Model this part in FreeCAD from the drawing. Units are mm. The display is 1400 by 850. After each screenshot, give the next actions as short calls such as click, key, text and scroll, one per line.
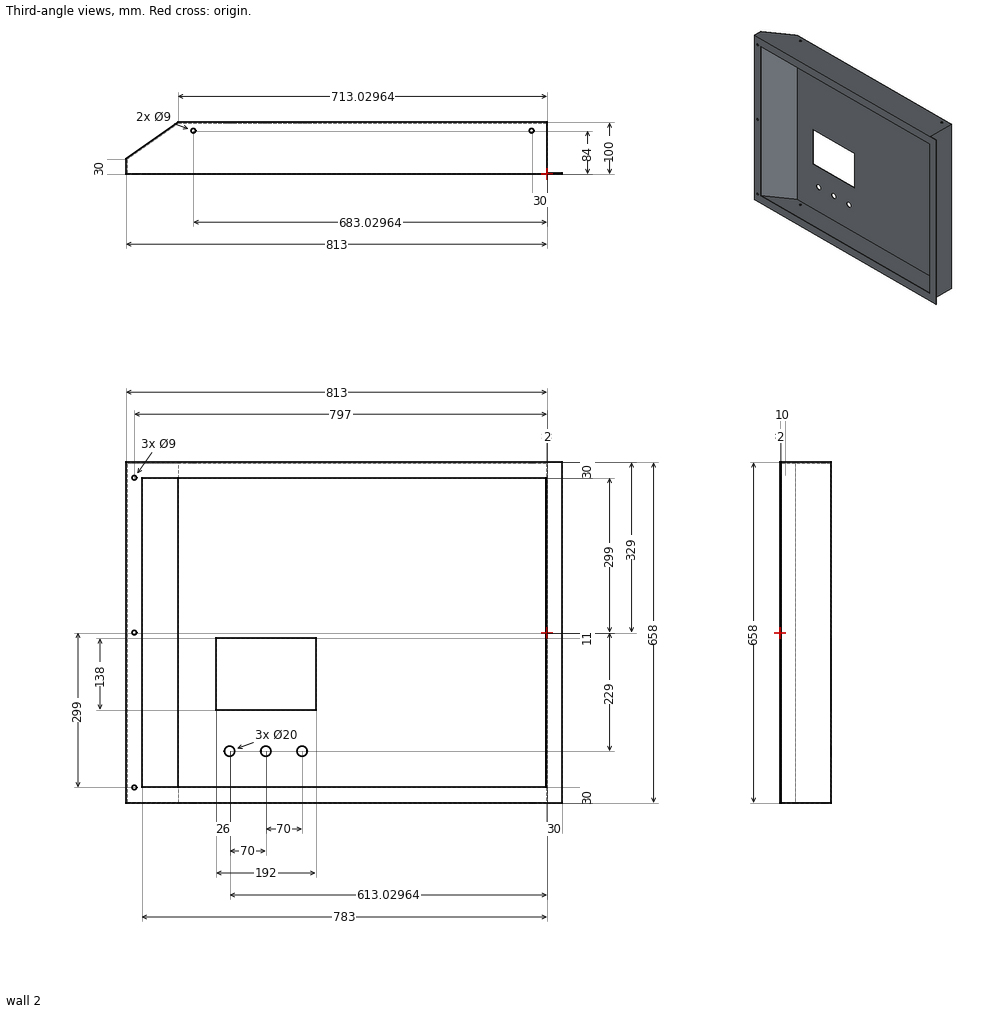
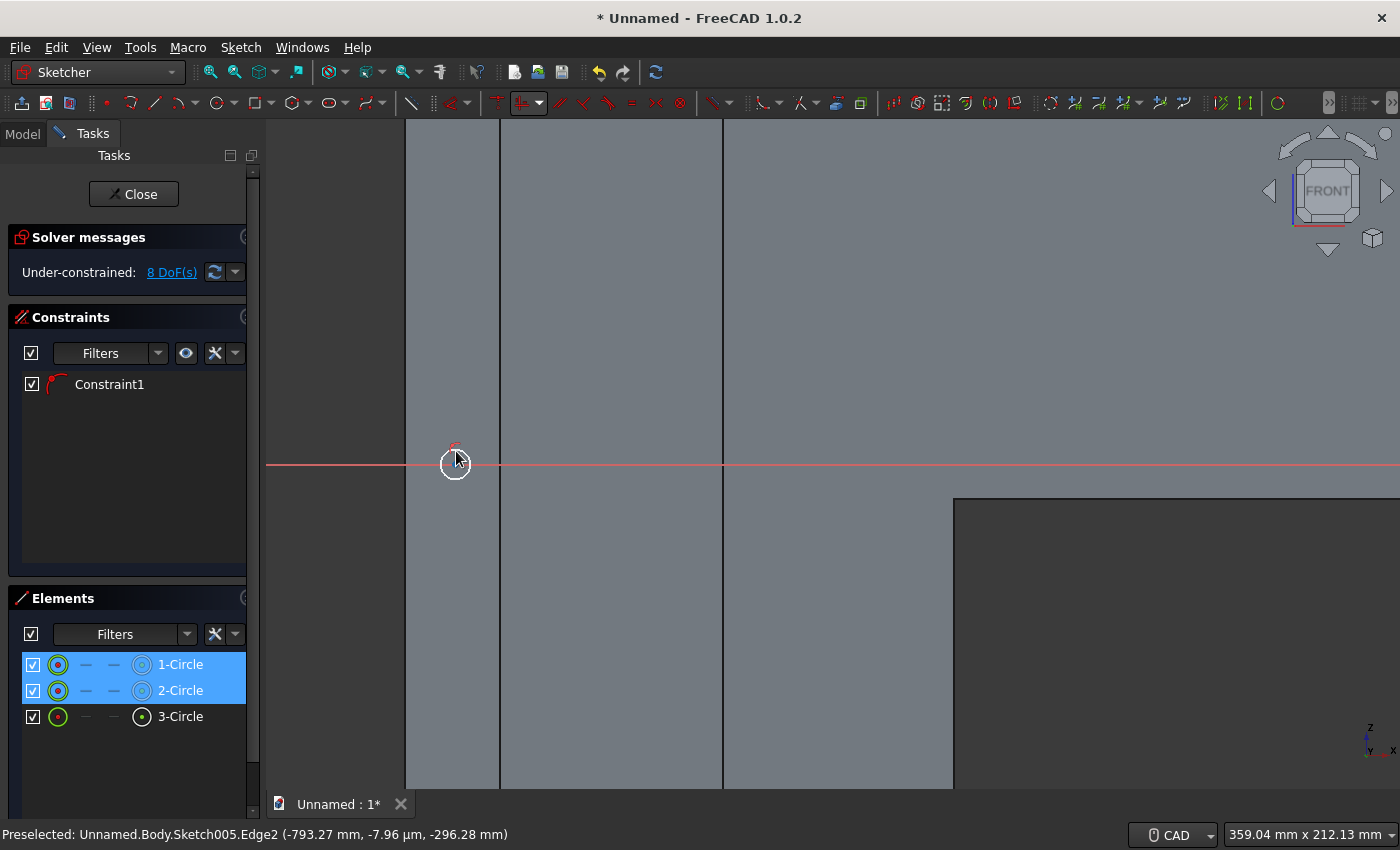
click(441, 464)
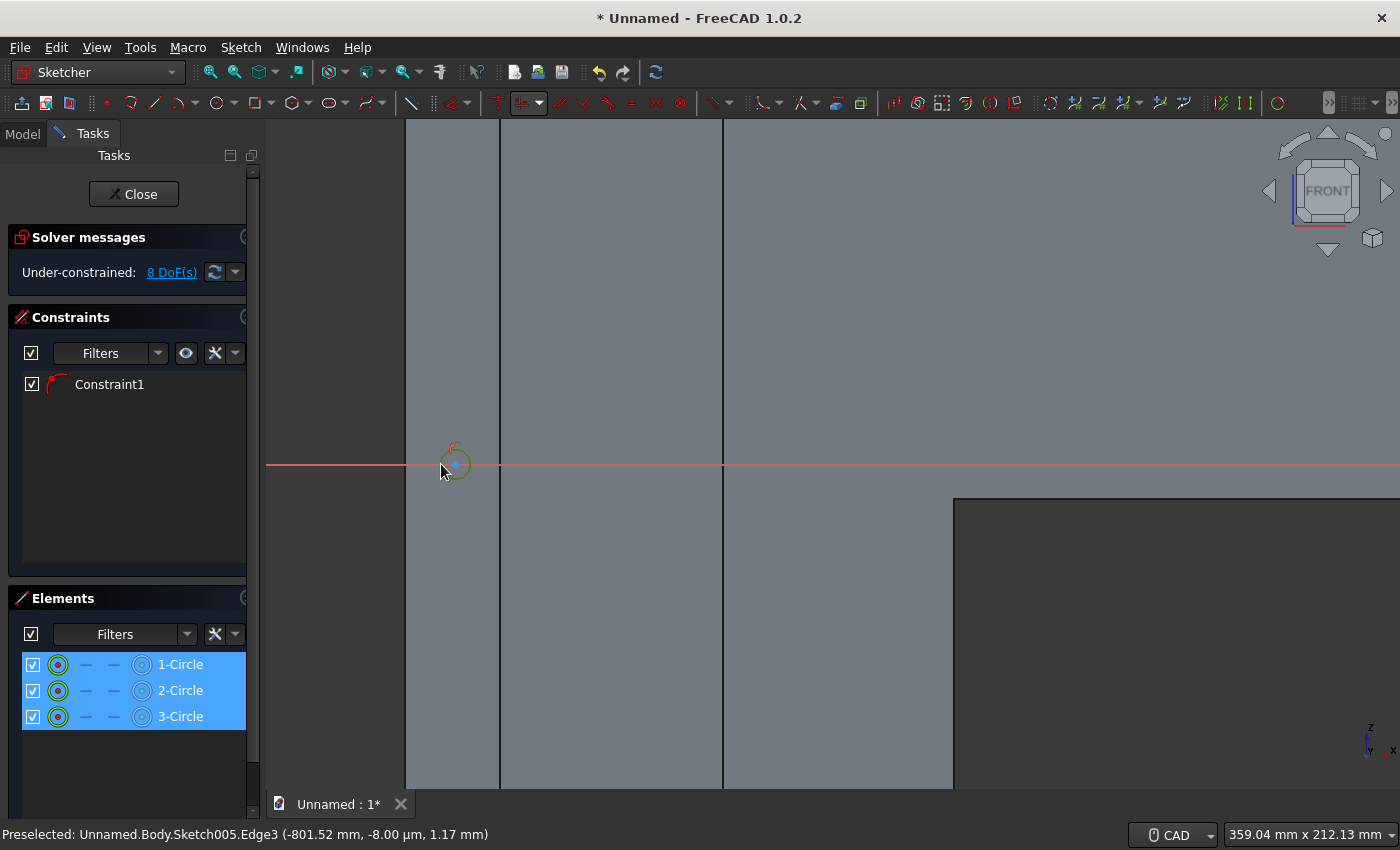
key(e)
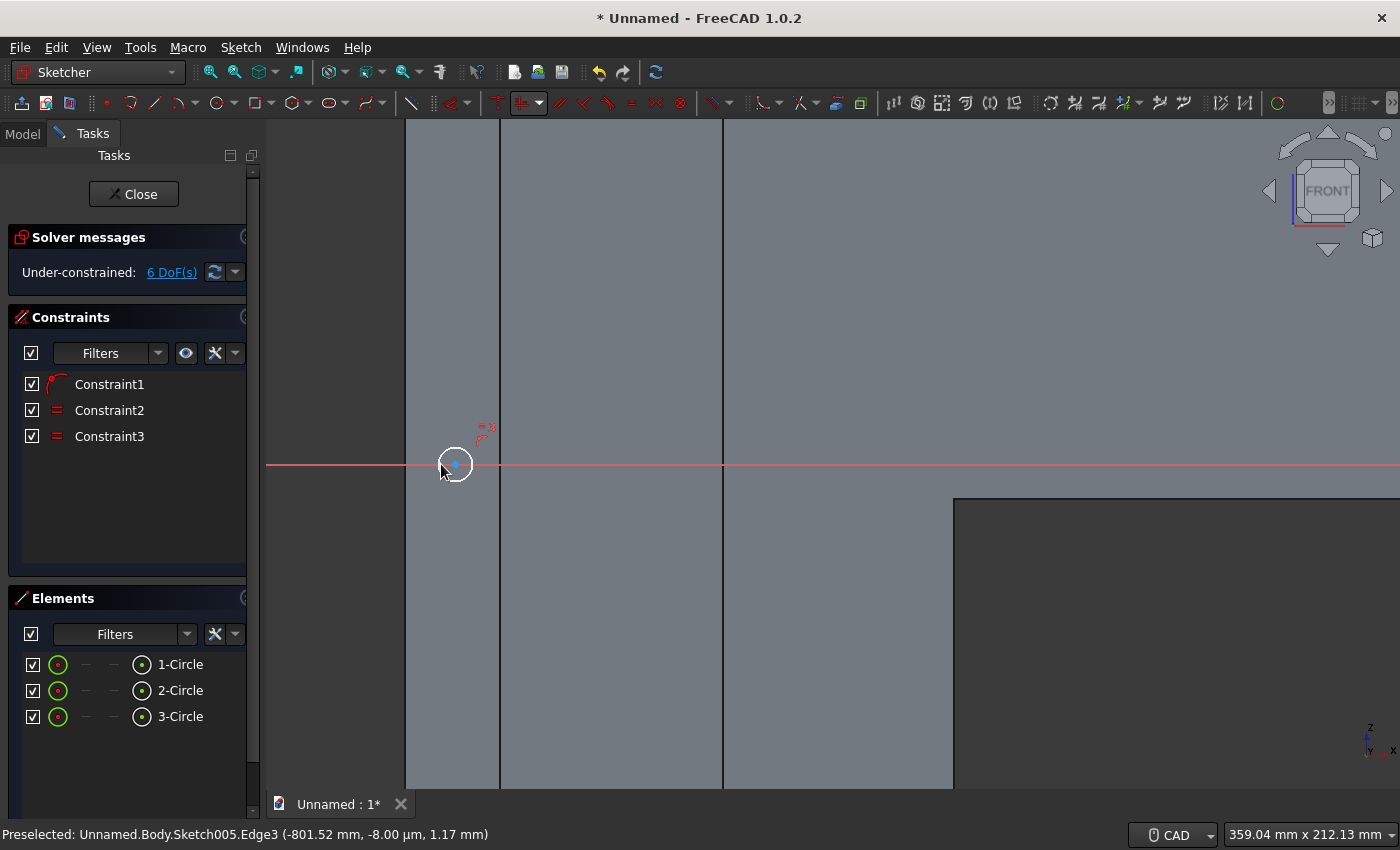
scroll(456, 451, down, 7)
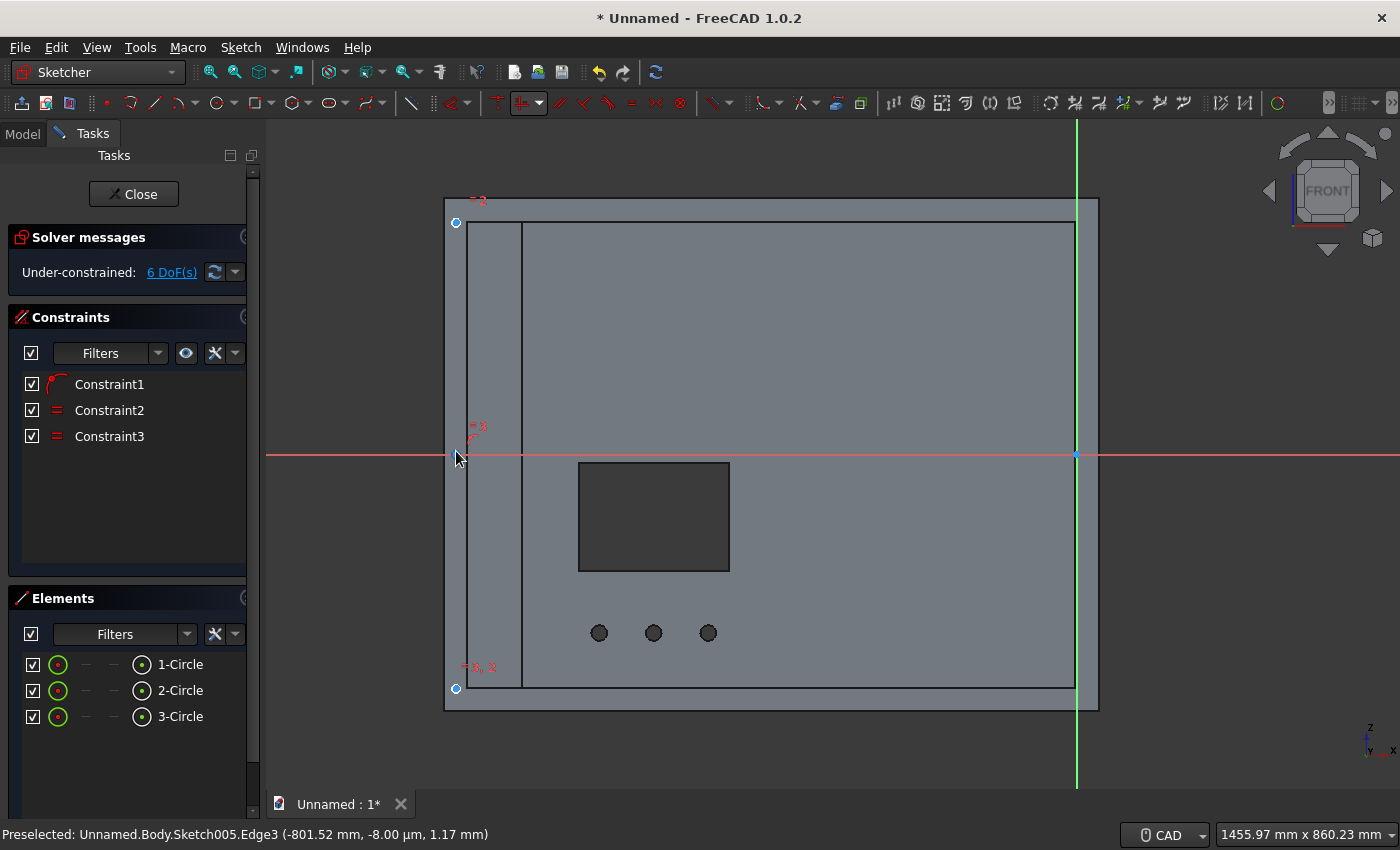
click(456, 223)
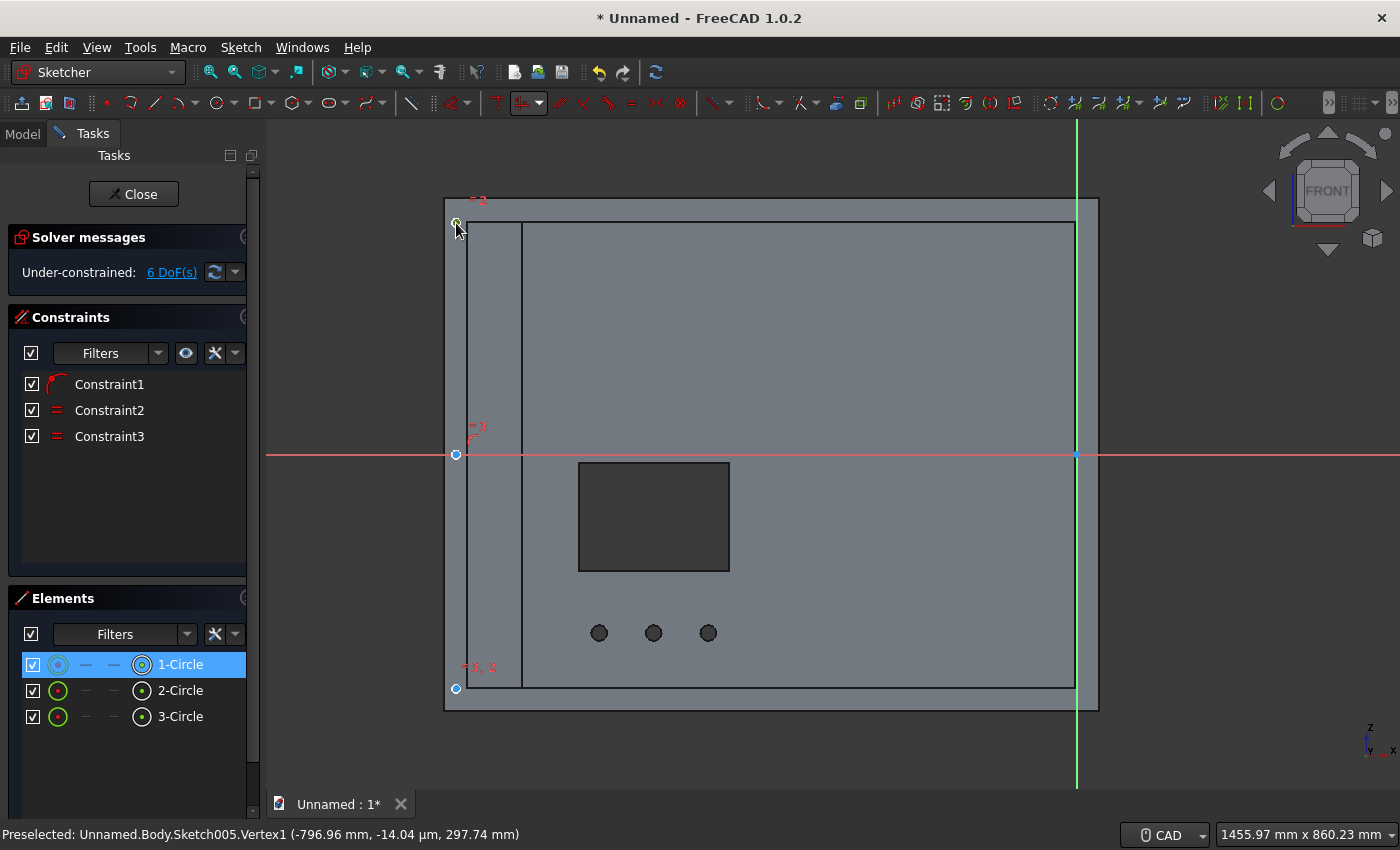
click(456, 689)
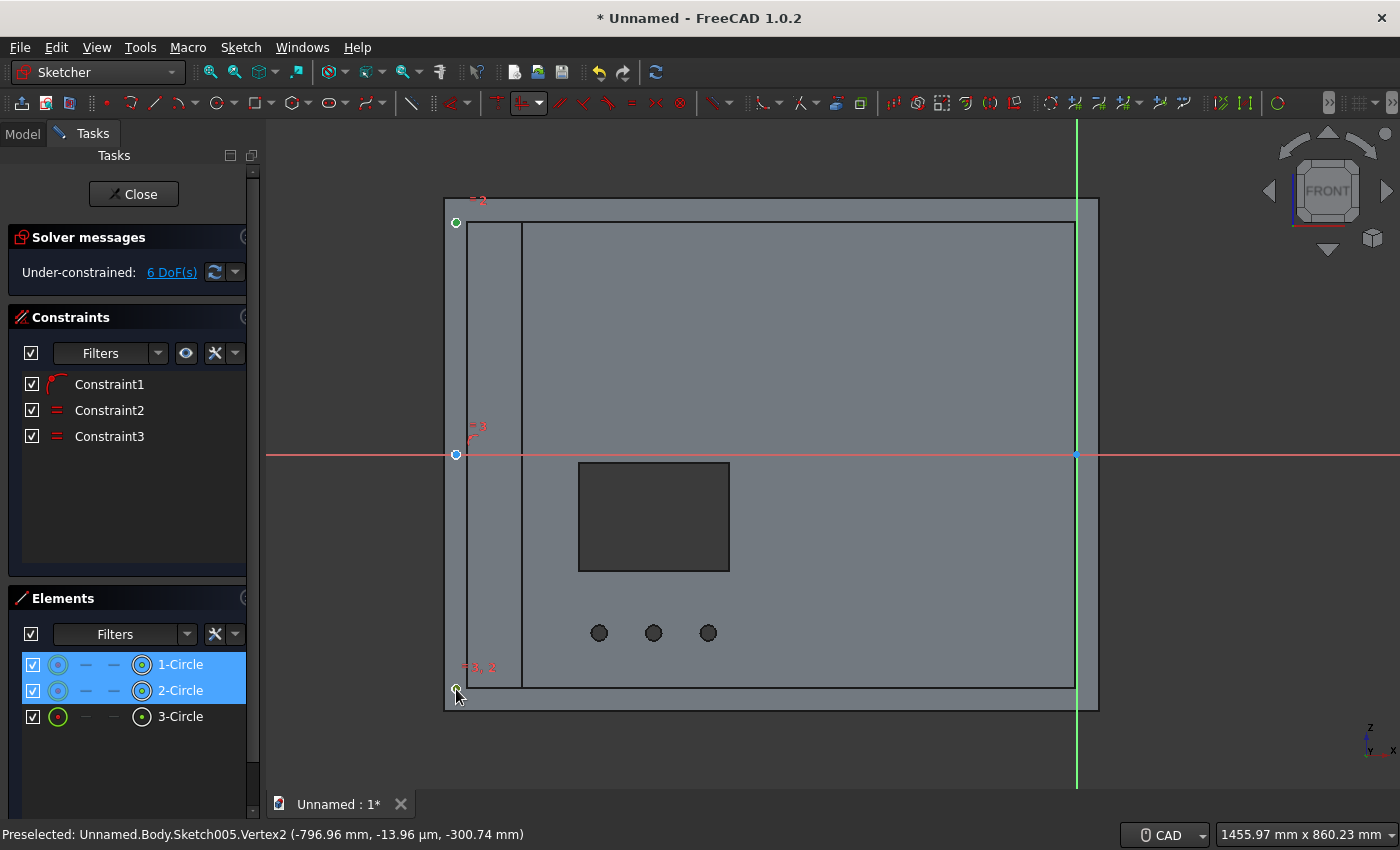
key(v)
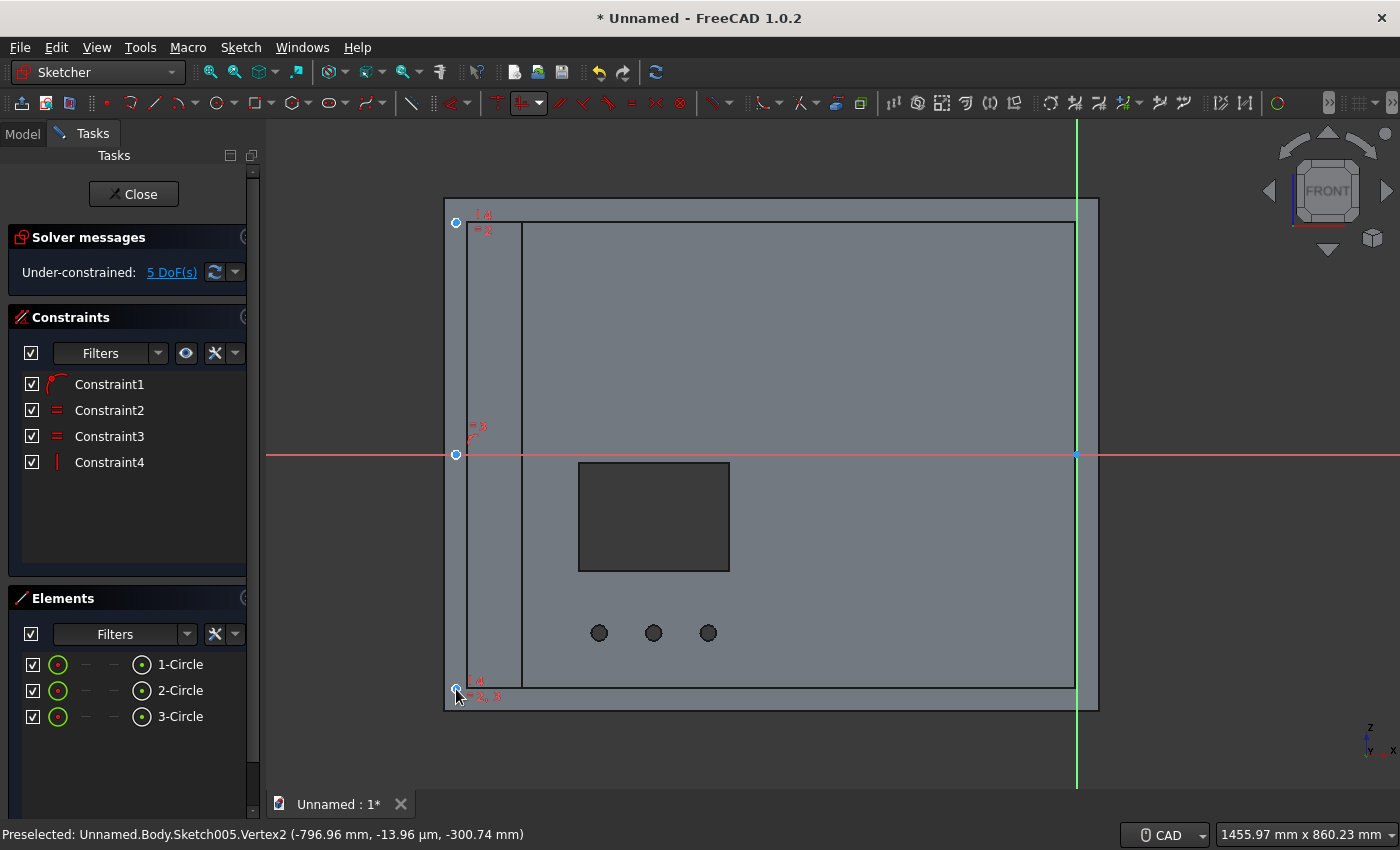
click(456, 223)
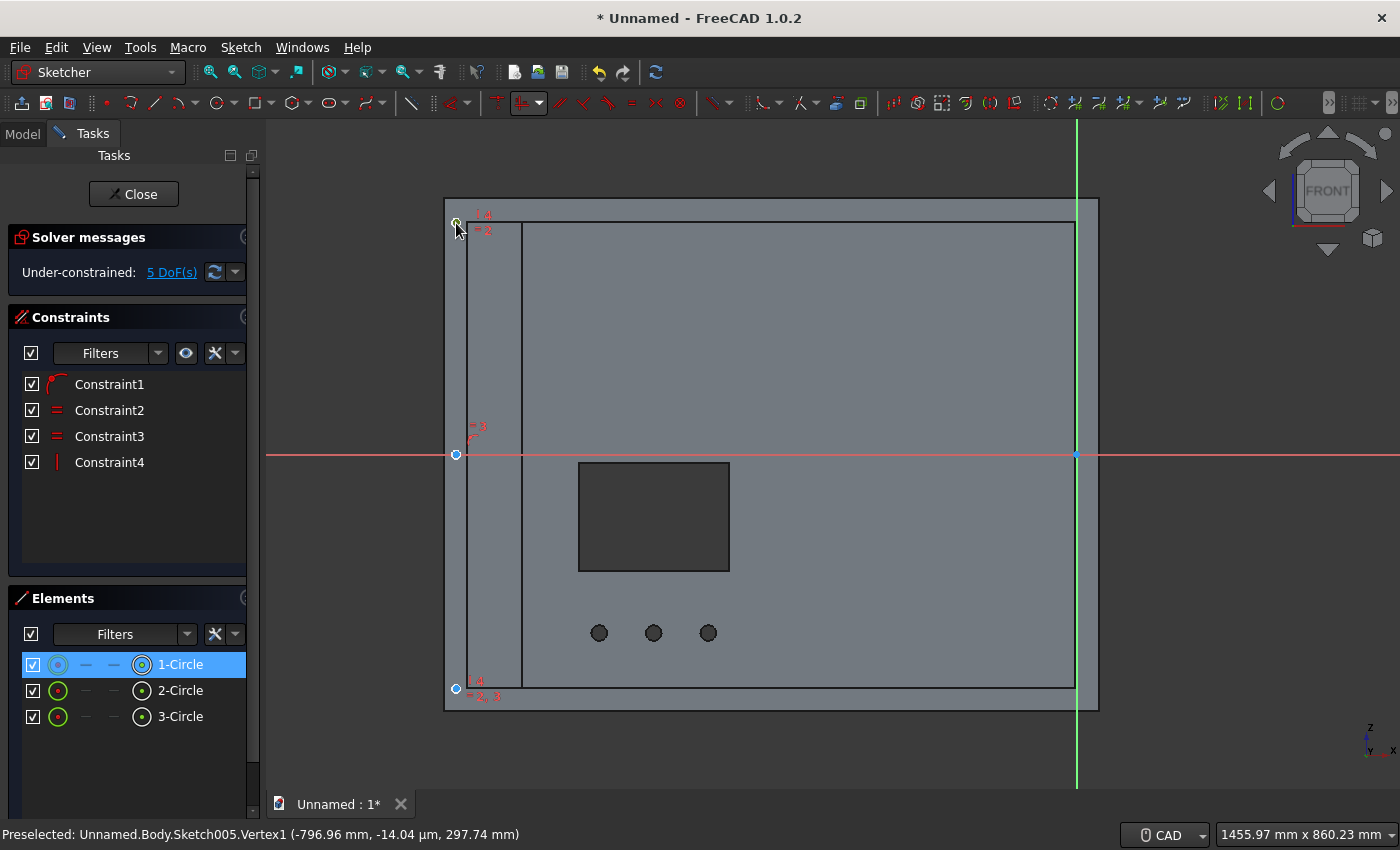
click(456, 455)